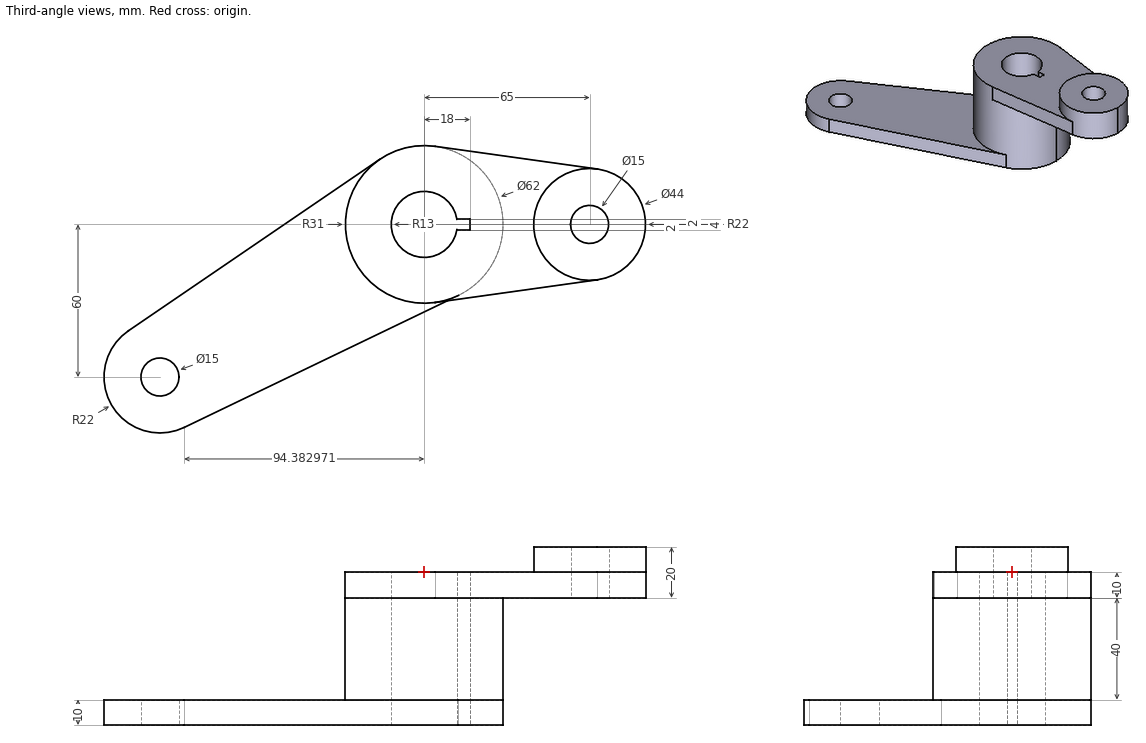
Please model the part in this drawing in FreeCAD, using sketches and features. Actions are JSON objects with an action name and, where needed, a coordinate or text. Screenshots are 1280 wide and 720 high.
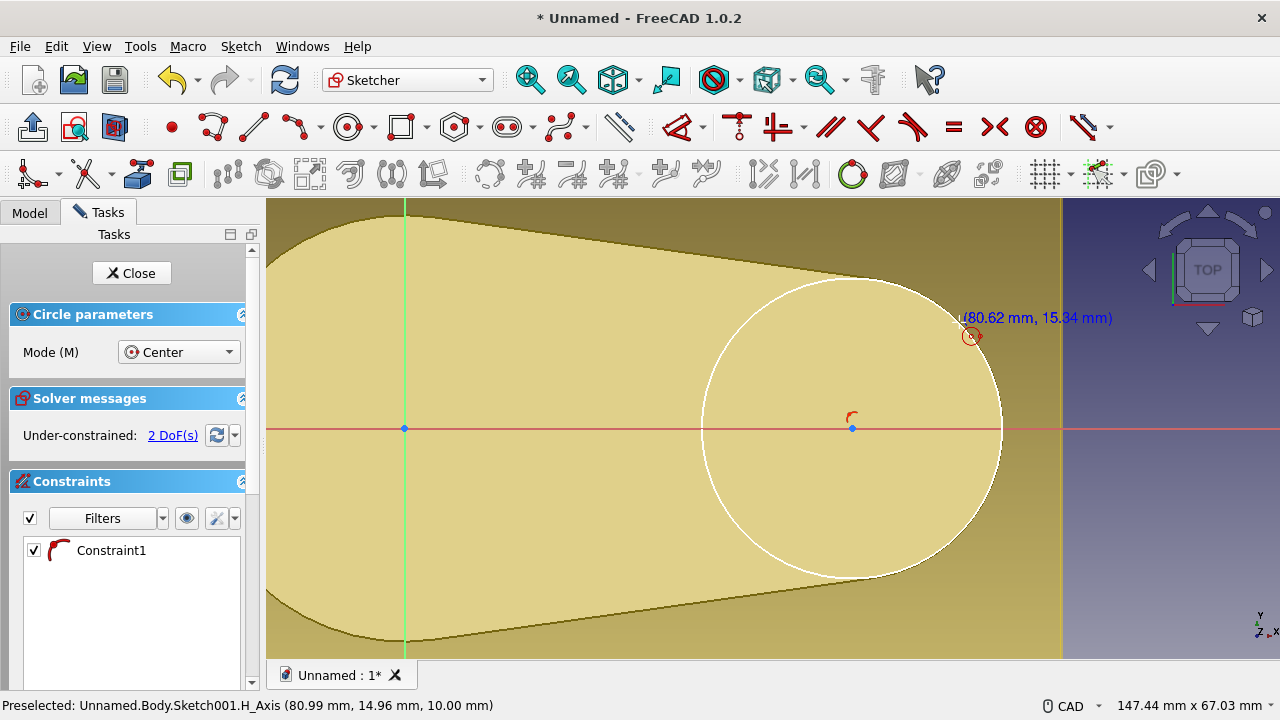
{"action": "left_click", "coordinate": [852, 428]}
{"action": "left_click", "coordinate": [888, 392]}
{"action": "key", "text": "Escape"}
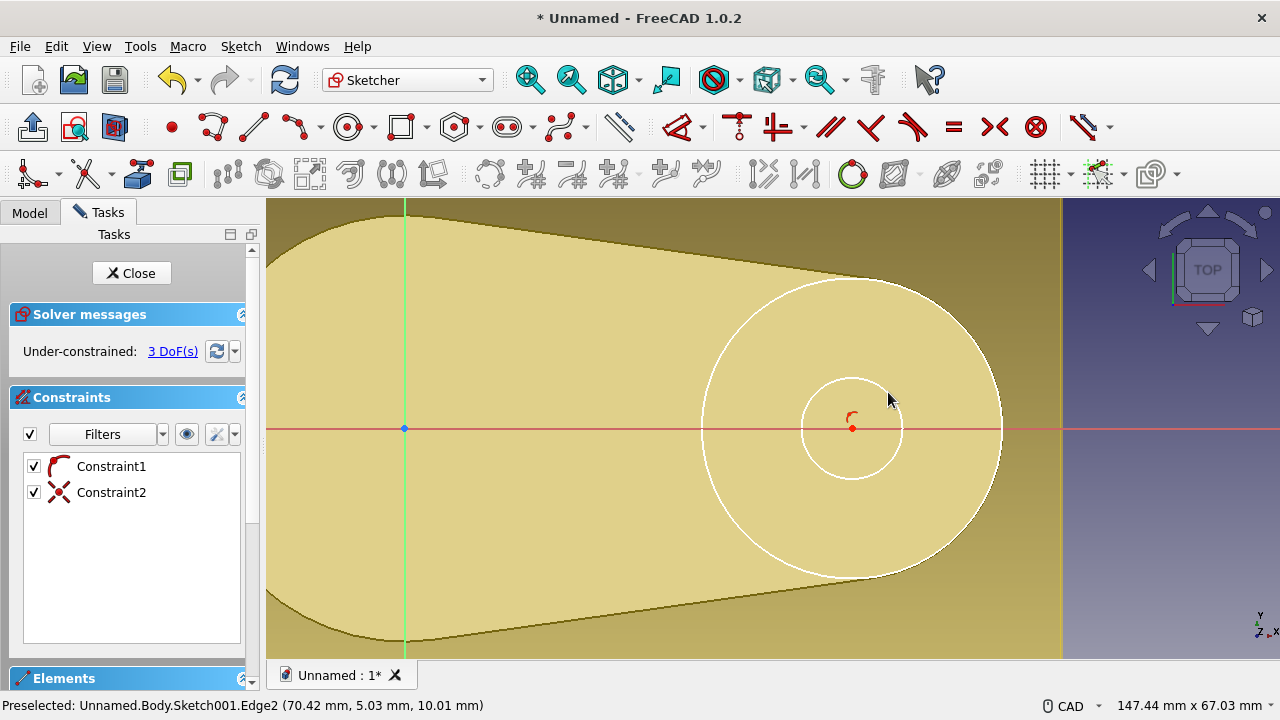
{"action": "key", "text": "d"}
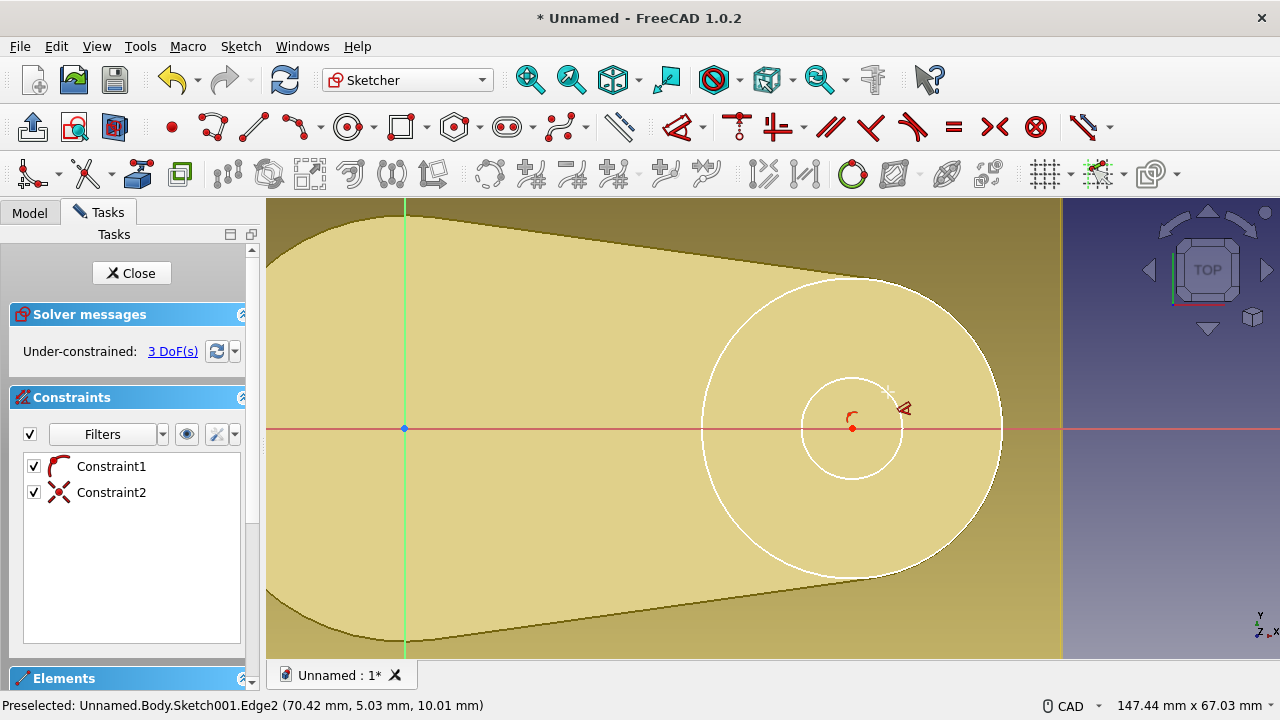
{"action": "left_click", "coordinate": [958, 322]}
{"action": "left_click", "coordinate": [981, 299]}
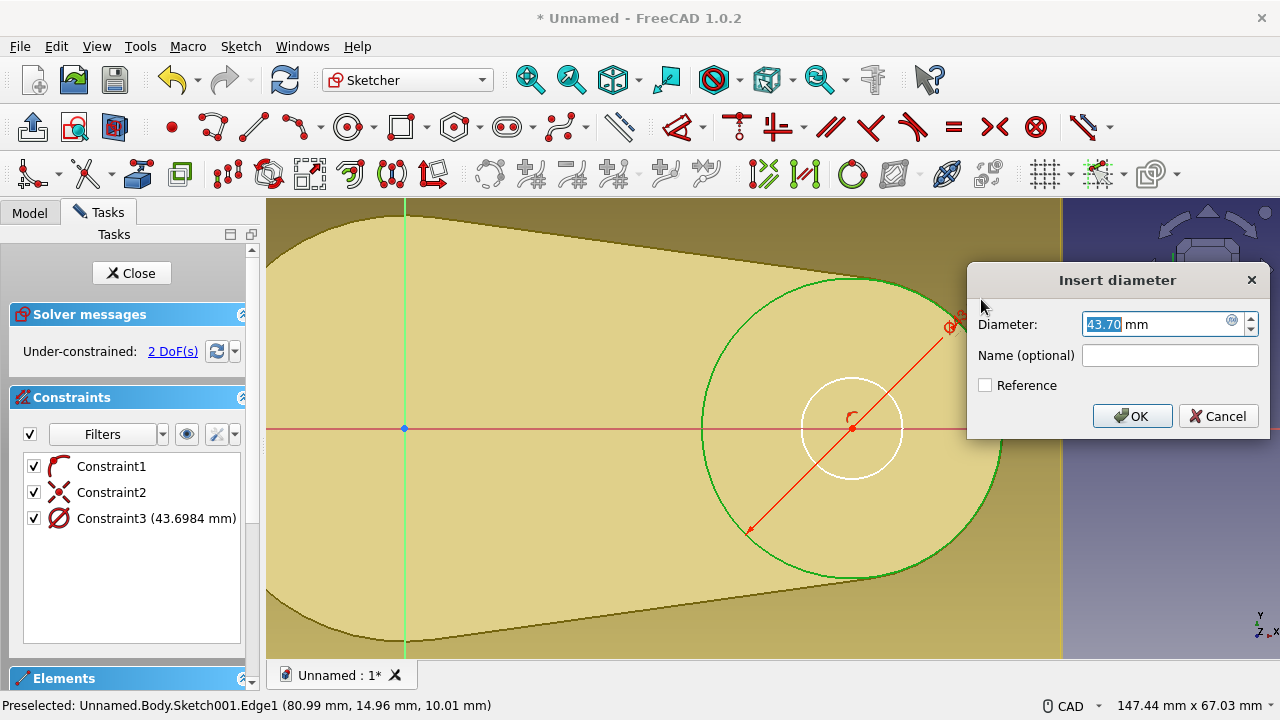
{"action": "type", "text": "44"}
{"action": "key", "text": "Return"}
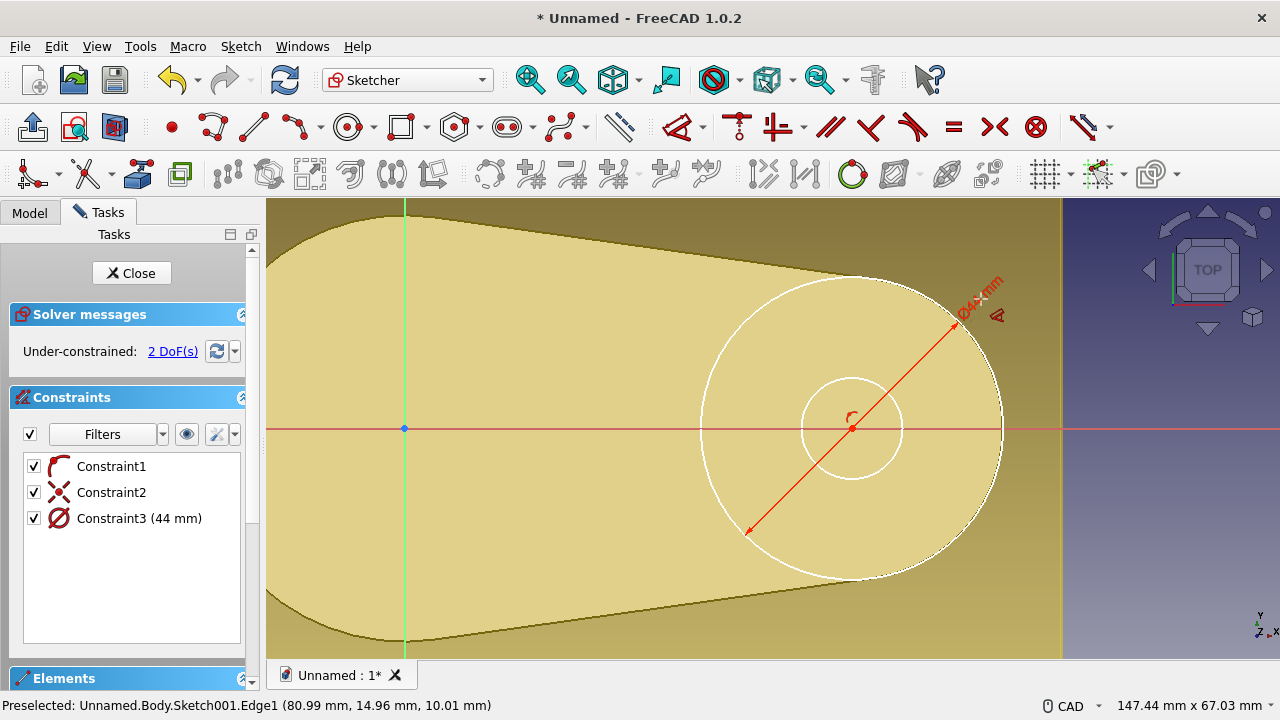
{"action": "left_click", "coordinate": [888, 393]}
{"action": "left_click", "coordinate": [911, 371]}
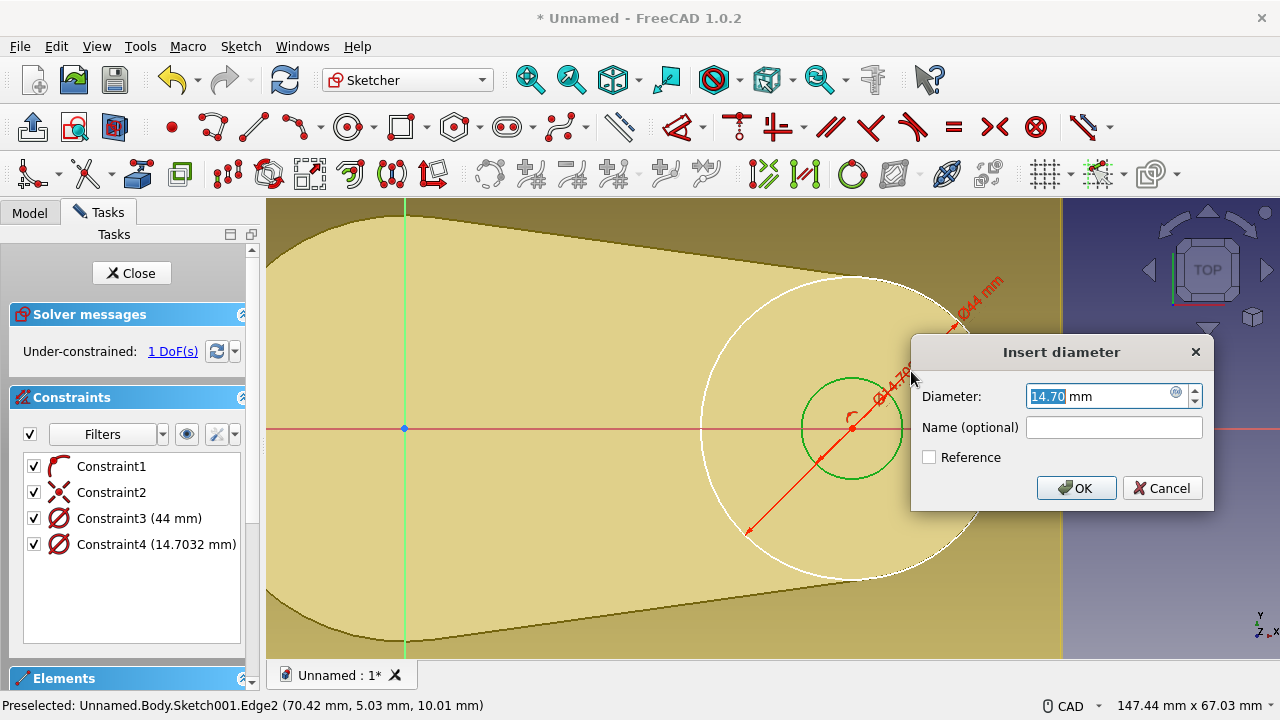
{"action": "type", "text": "15"}
{"action": "key", "text": "Return"}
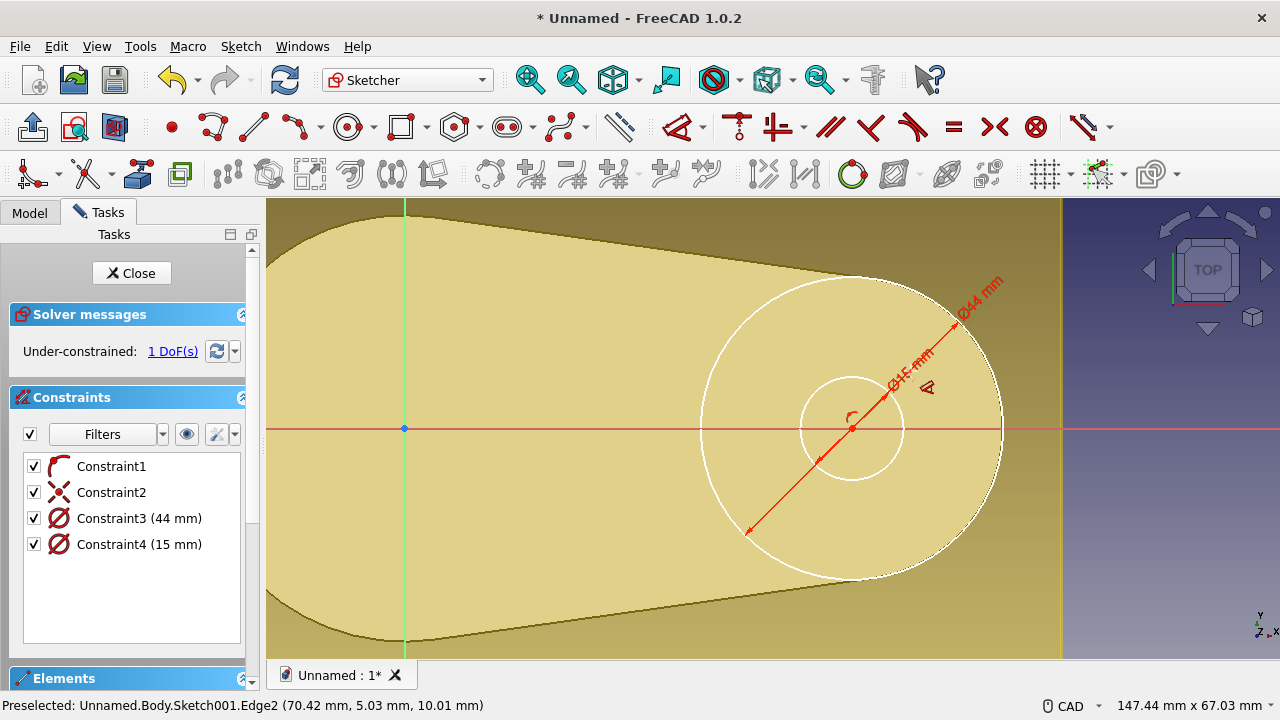
{"action": "left_click", "coordinate": [852, 428]}
{"action": "left_click", "coordinate": [628, 462]}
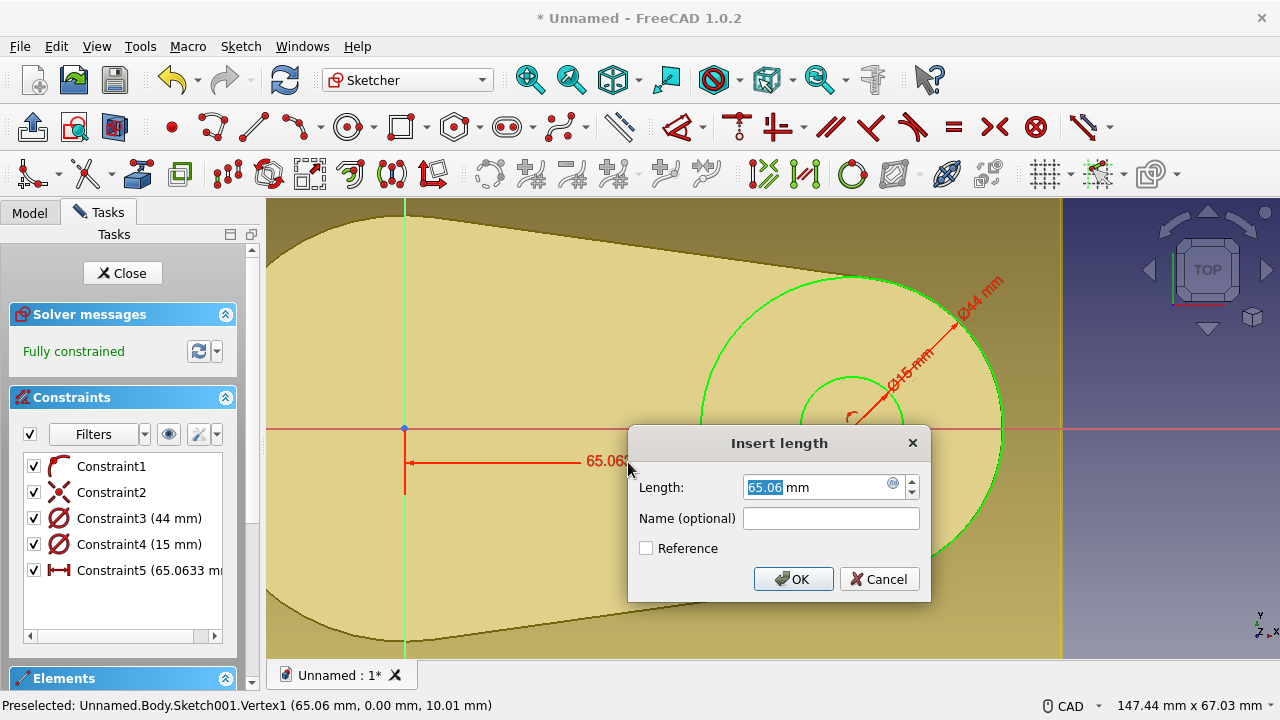
{"action": "type", "text": "65"}
{"action": "key", "text": "Return"}
{"action": "key", "text": "Escape"}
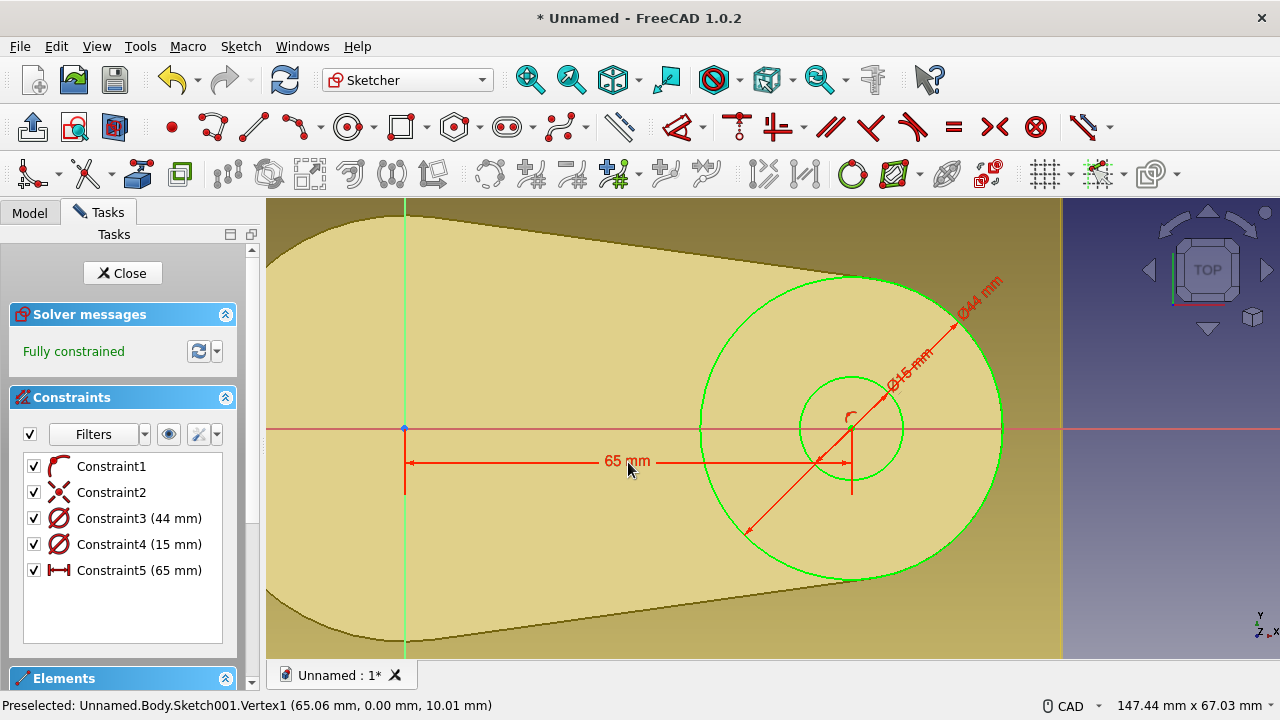
{"action": "left_click", "coordinate": [123, 273]}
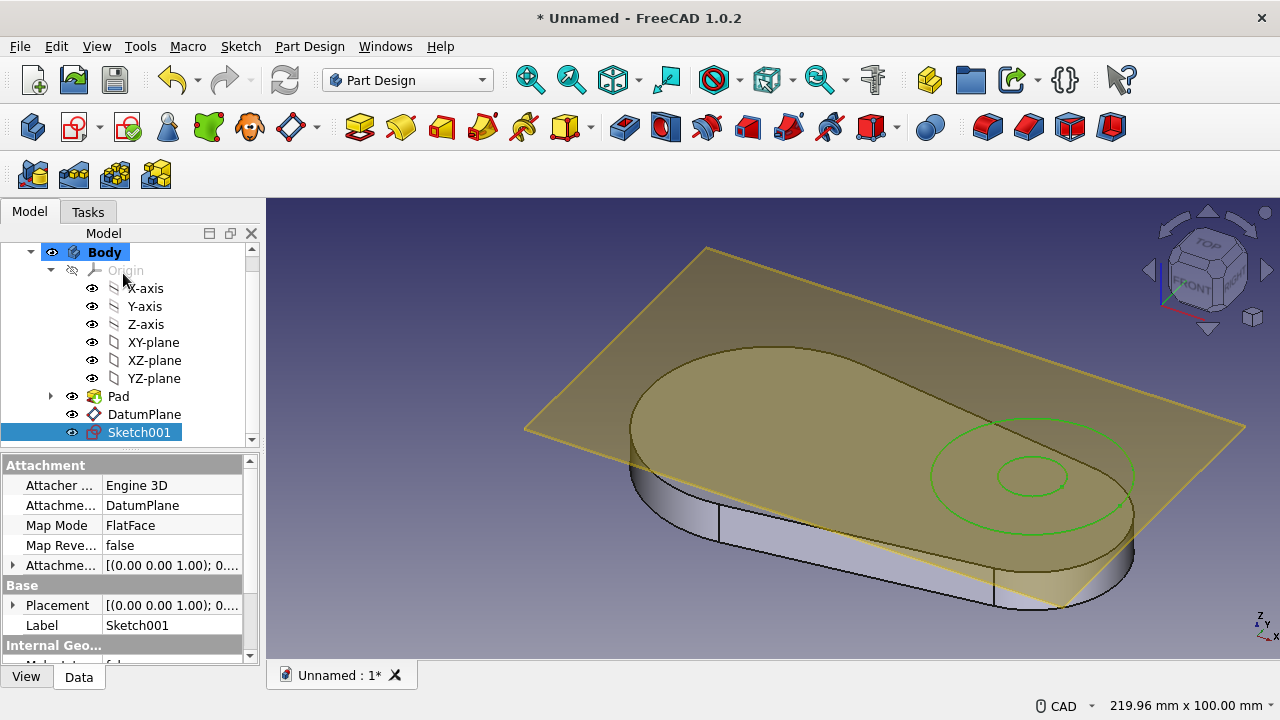
{"action": "left_click", "coordinate": [360, 128]}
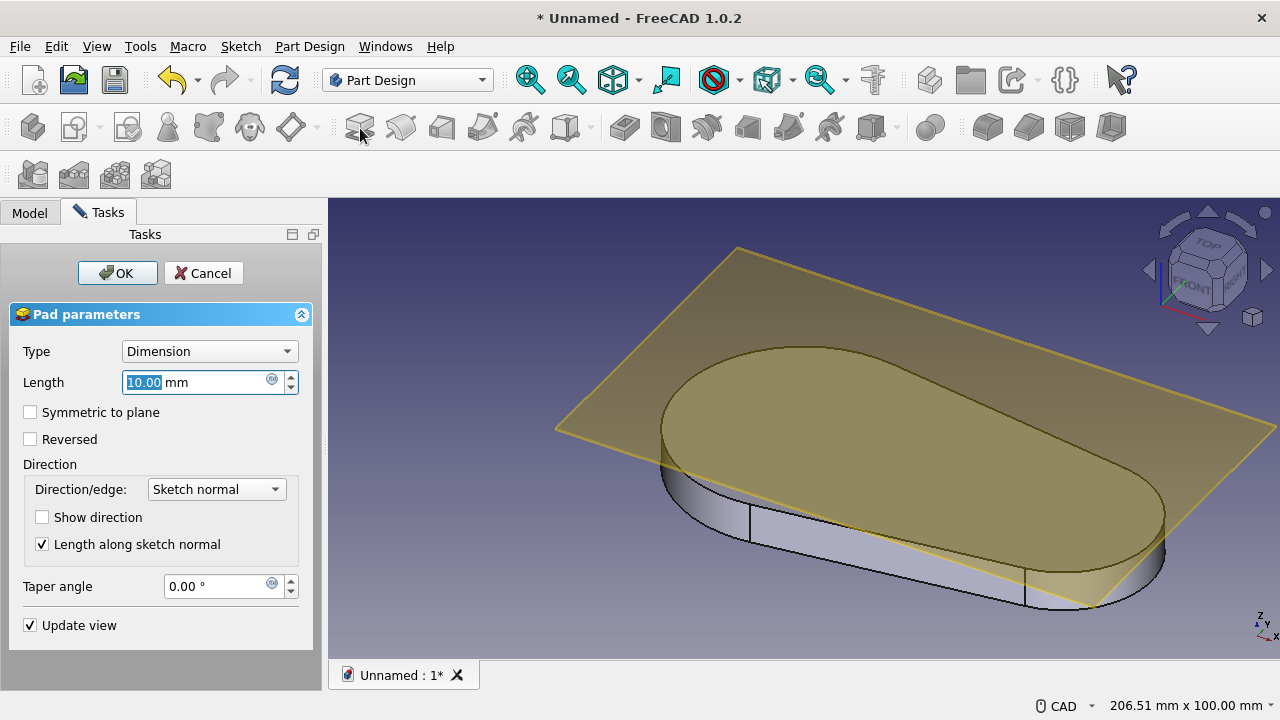
{"action": "type", "text": "20"}
{"action": "key", "text": "Tab"}